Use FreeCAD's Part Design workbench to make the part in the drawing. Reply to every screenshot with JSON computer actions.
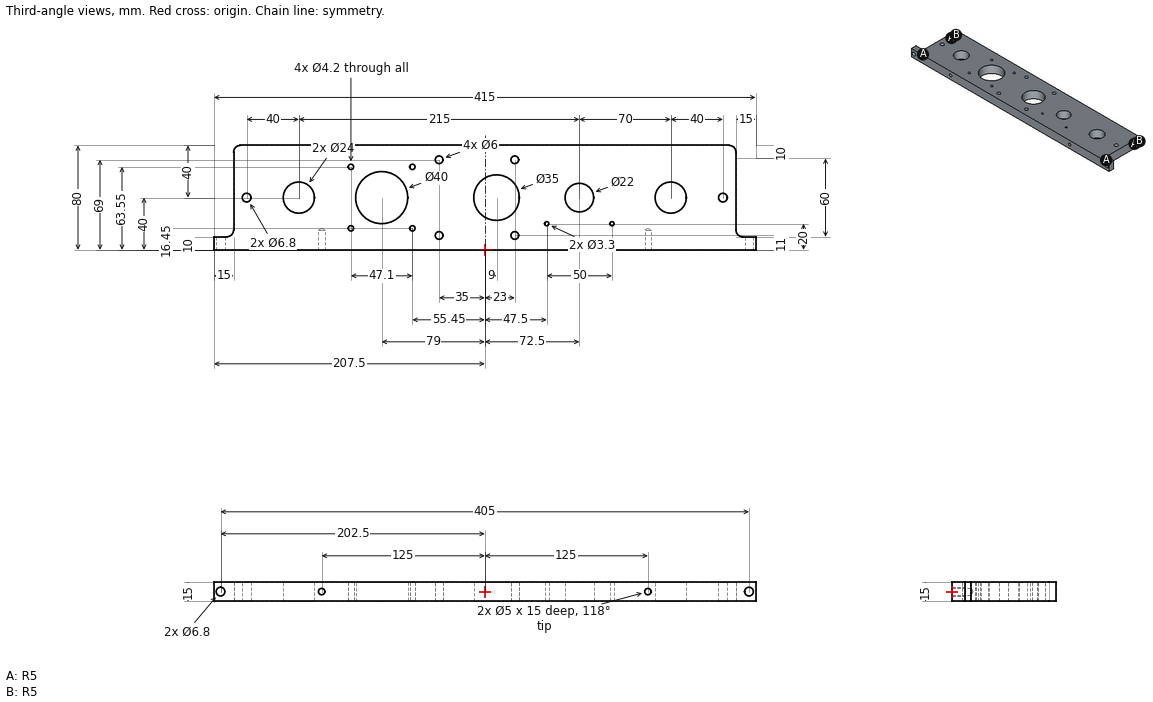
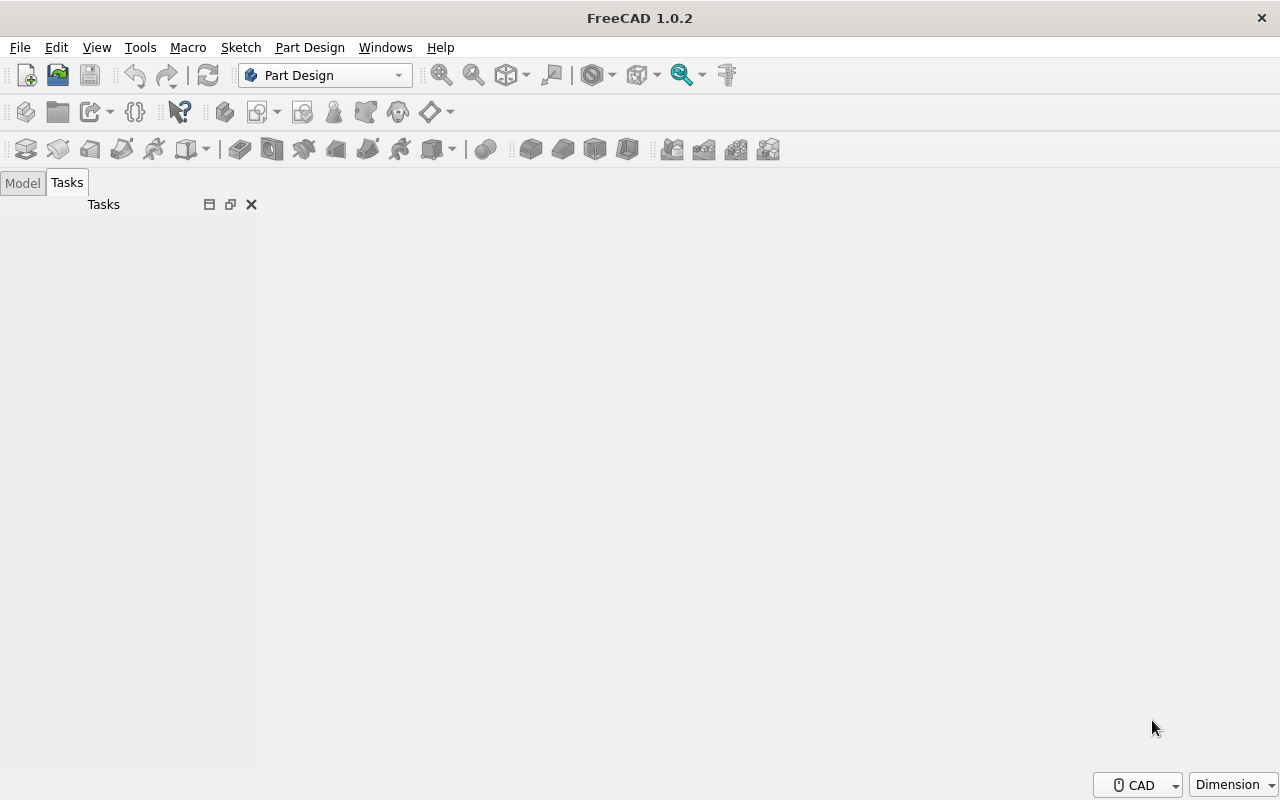
{"action": "left_click", "coordinate": [26, 76]}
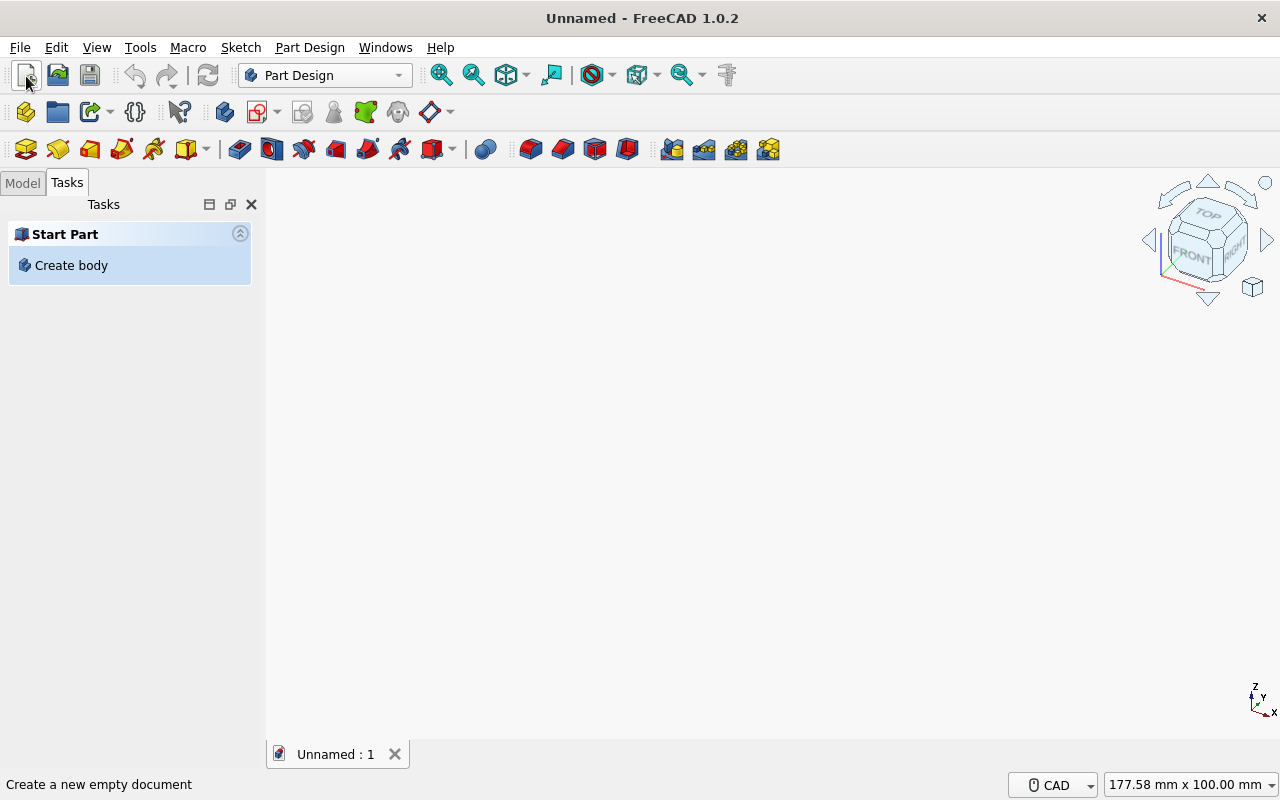
{"action": "left_click", "coordinate": [258, 112]}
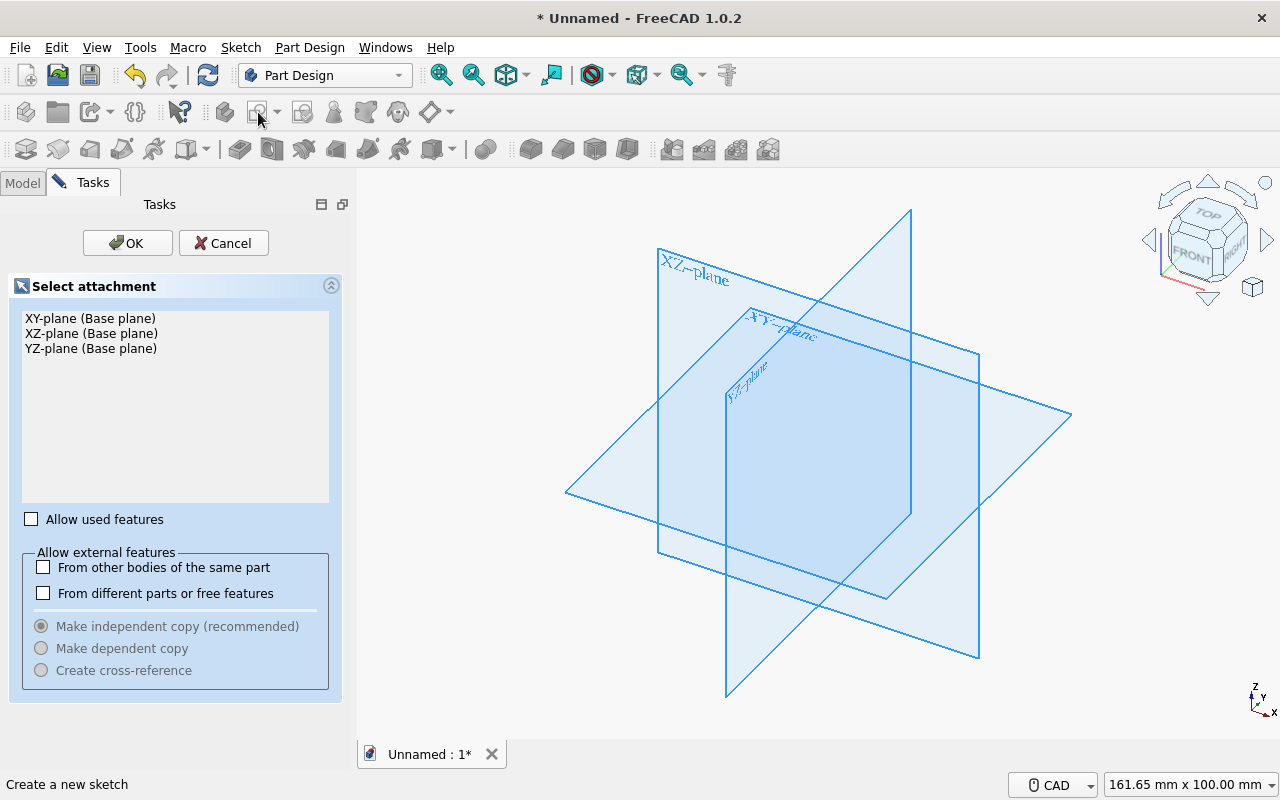
{"action": "left_click", "coordinate": [82, 318]}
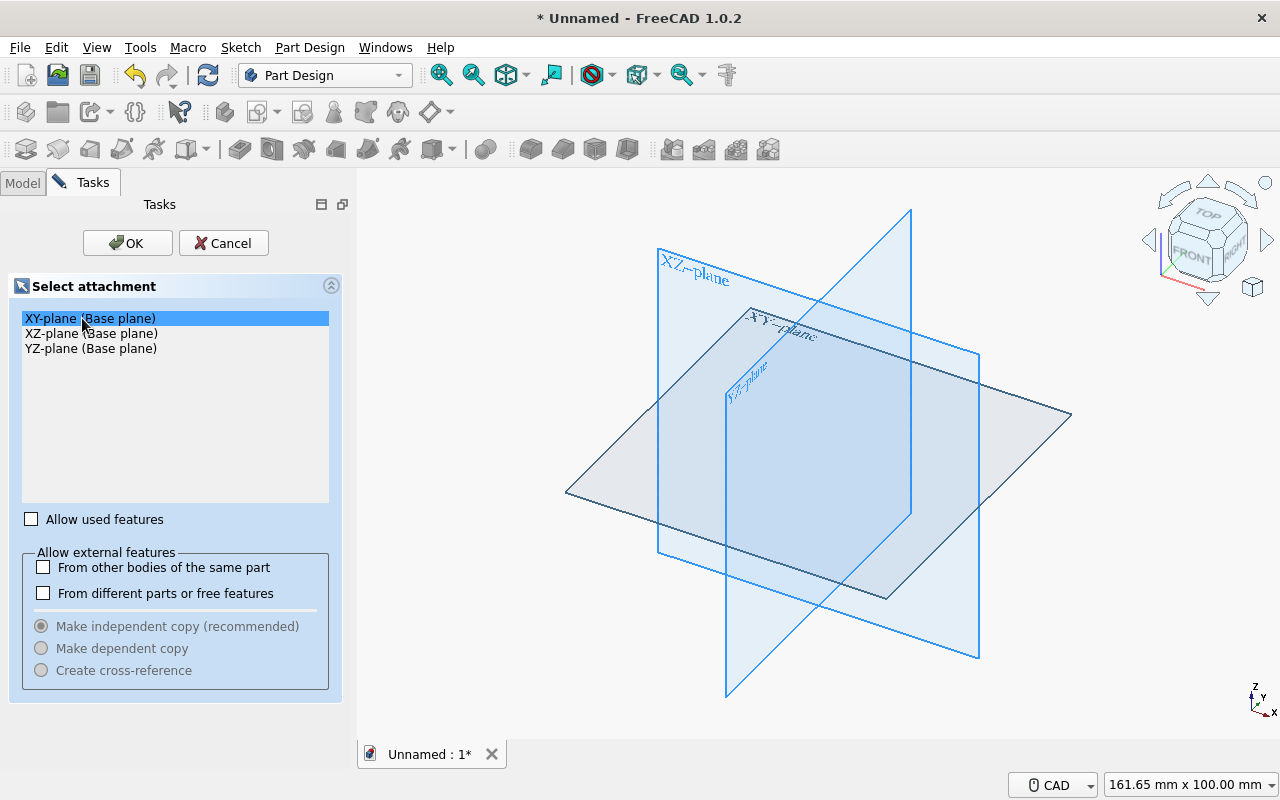
{"action": "left_click", "coordinate": [128, 243]}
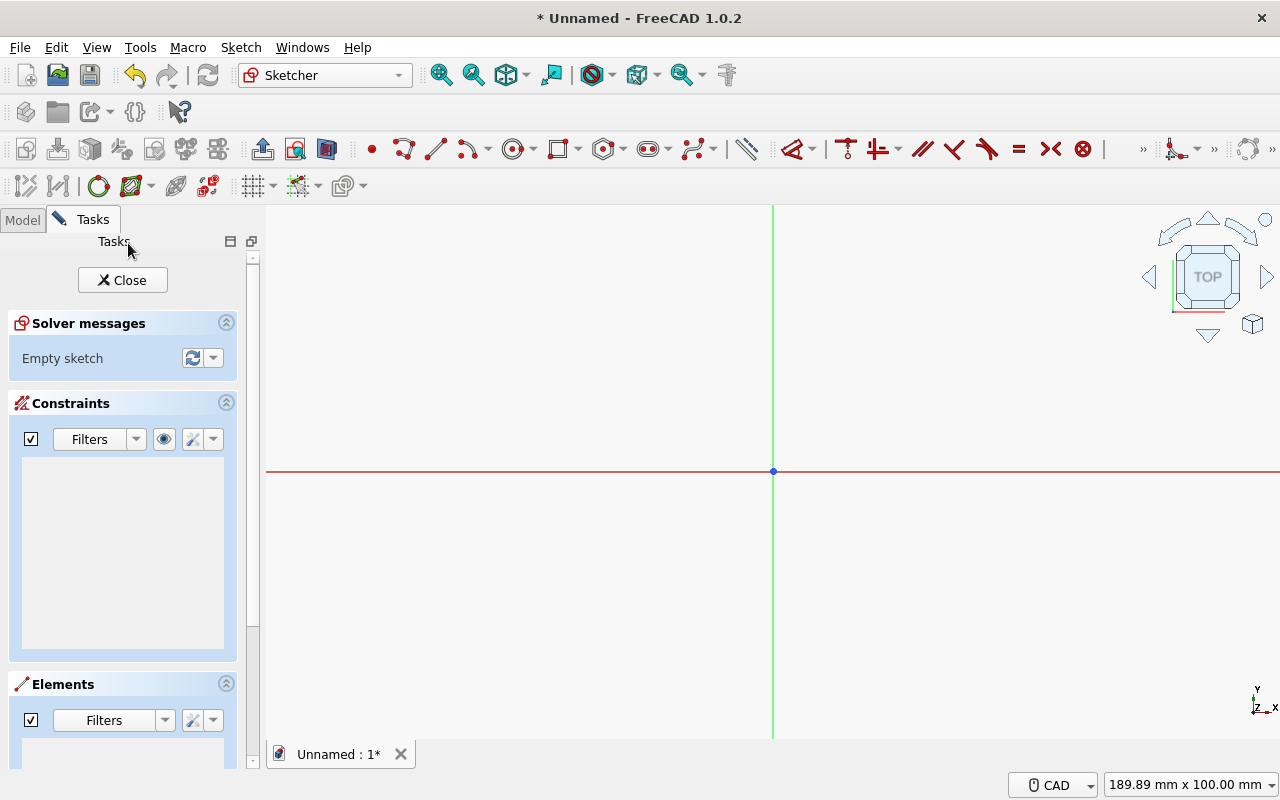
{"action": "scroll", "coordinate": [682, 542], "scroll_direction": "down", "scroll_amount": 7}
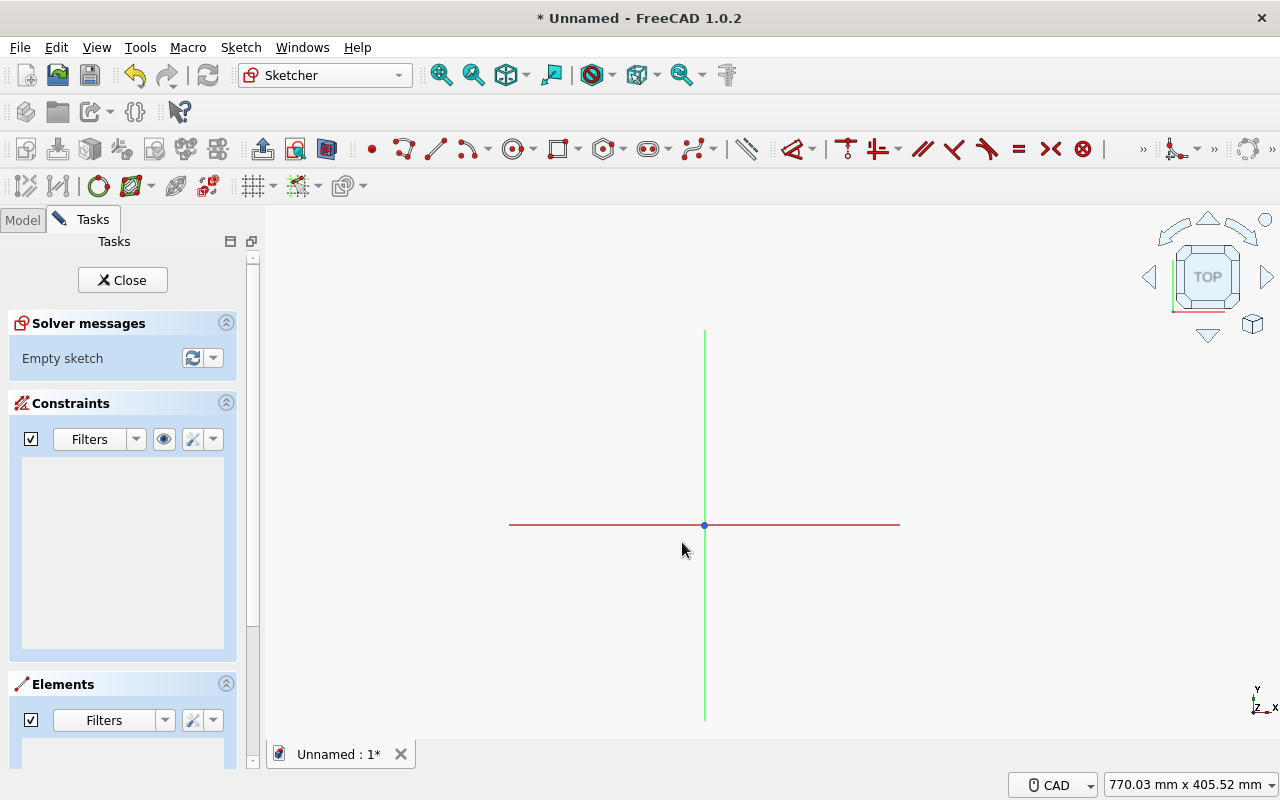
{"action": "left_click", "coordinate": [404, 150]}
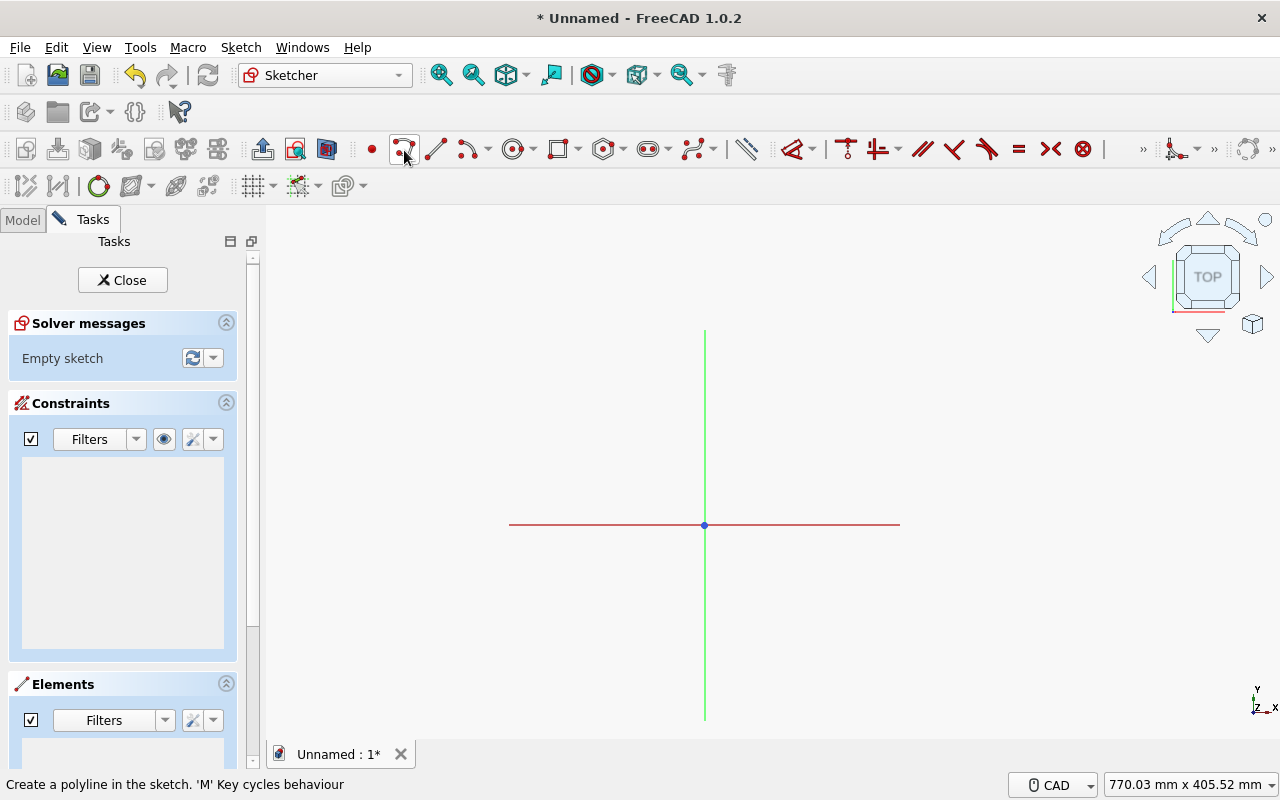
{"action": "left_click", "coordinate": [958, 512]}
{"action": "left_click", "coordinate": [958, 433]}
{"action": "left_click", "coordinate": [978, 433]}
{"action": "left_click", "coordinate": [978, 420]}
{"action": "left_click", "coordinate": [432, 420]}
{"action": "left_click", "coordinate": [432, 433]}
{"action": "left_click", "coordinate": [451, 433]}
{"action": "left_click", "coordinate": [451, 512]}
{"action": "left_click", "coordinate": [432, 512]}
{"action": "left_click", "coordinate": [432, 525]}
{"action": "left_click", "coordinate": [978, 516]}
{"action": "left_click", "coordinate": [978, 512]}
{"action": "left_click", "coordinate": [958, 513]}
{"action": "key", "text": "Escape"}
{"action": "key", "text": "Escape"}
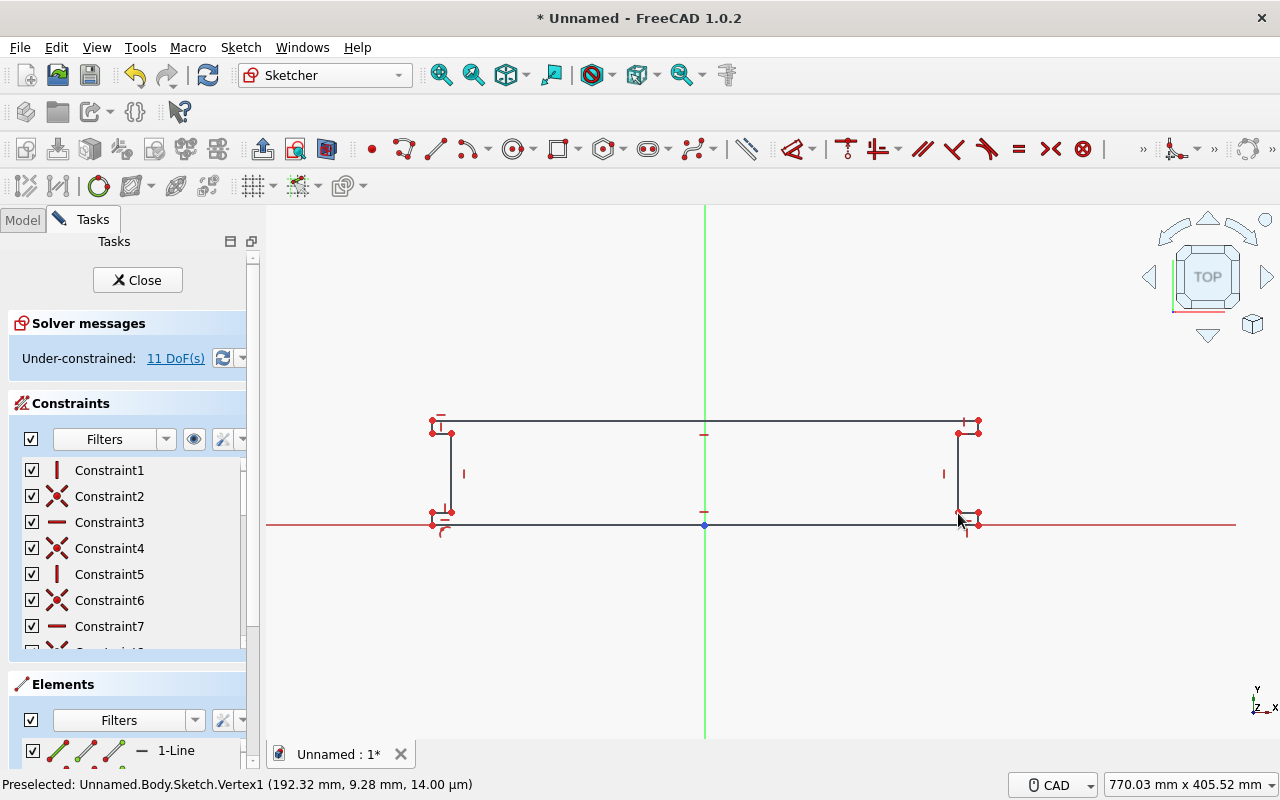
{"action": "left_click", "coordinate": [978, 434]}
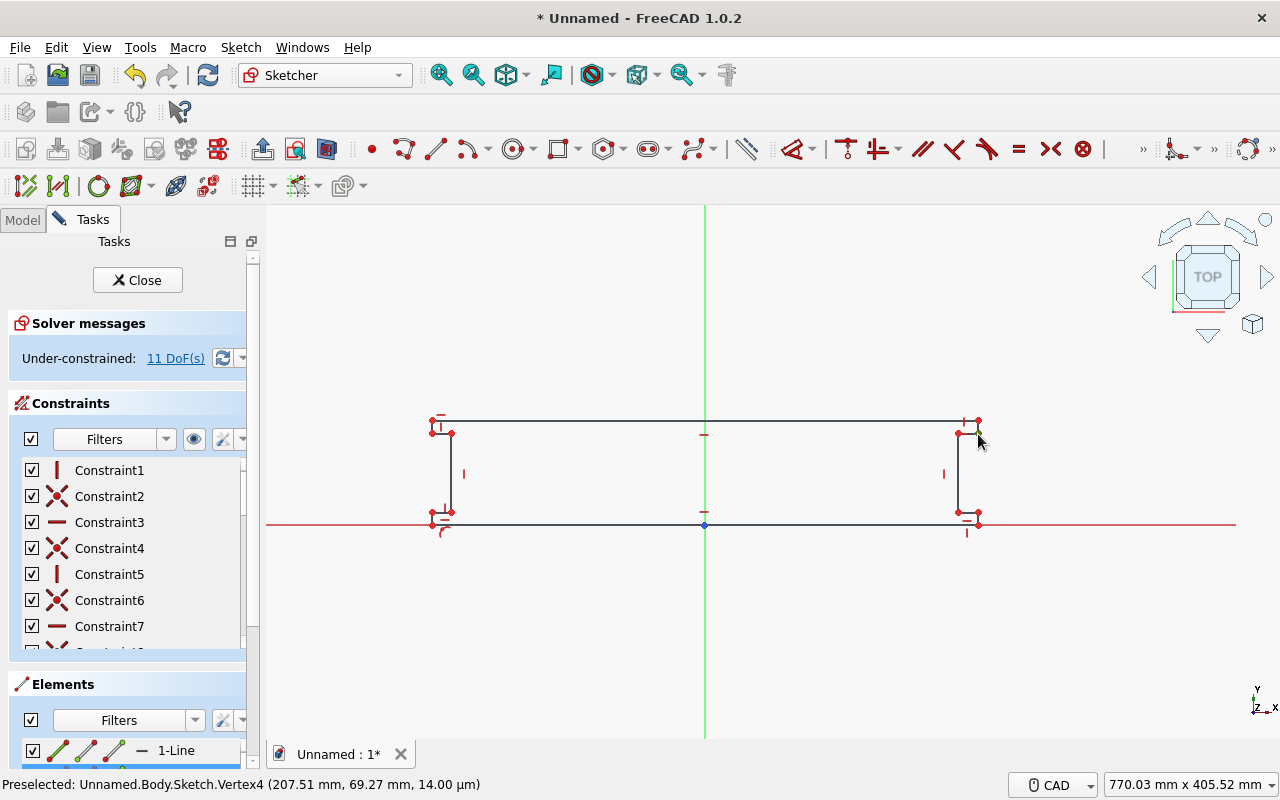
{"action": "left_click", "coordinate": [432, 434]}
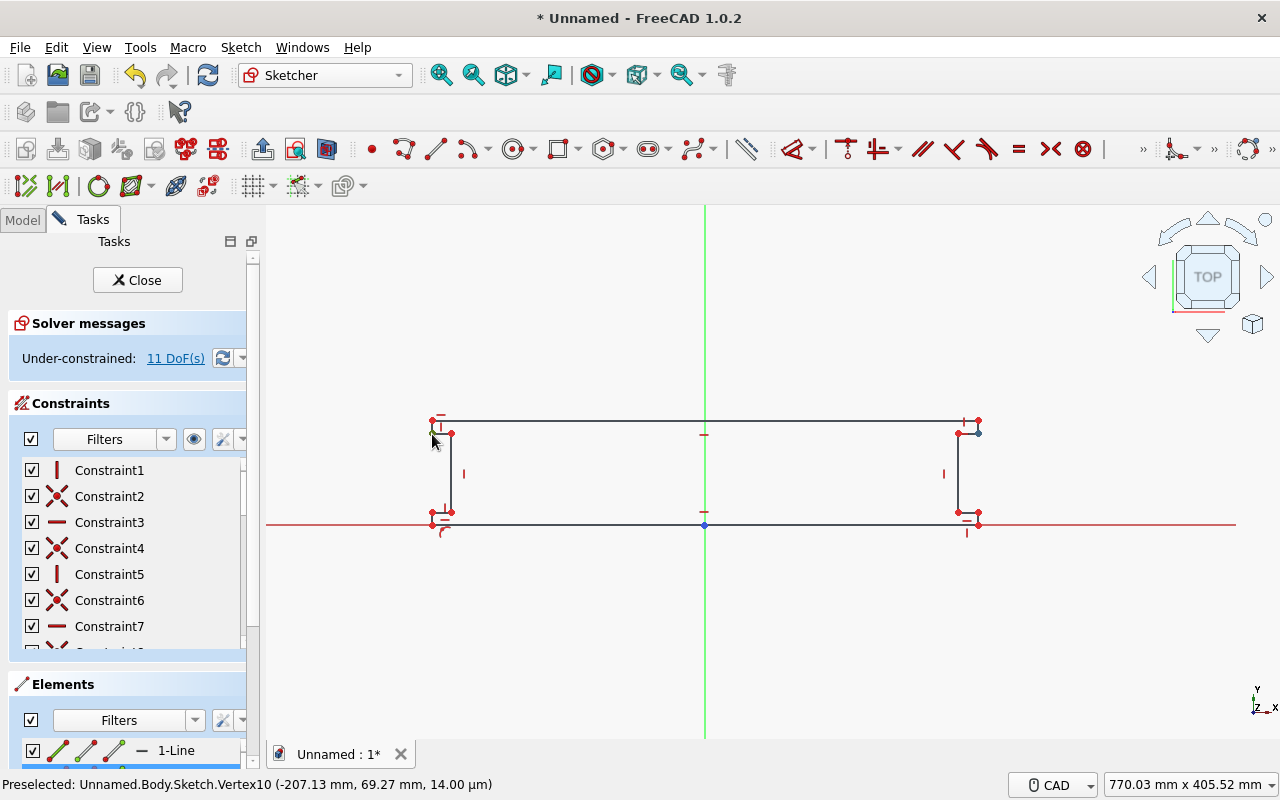
{"action": "left_click", "coordinate": [705, 677]}